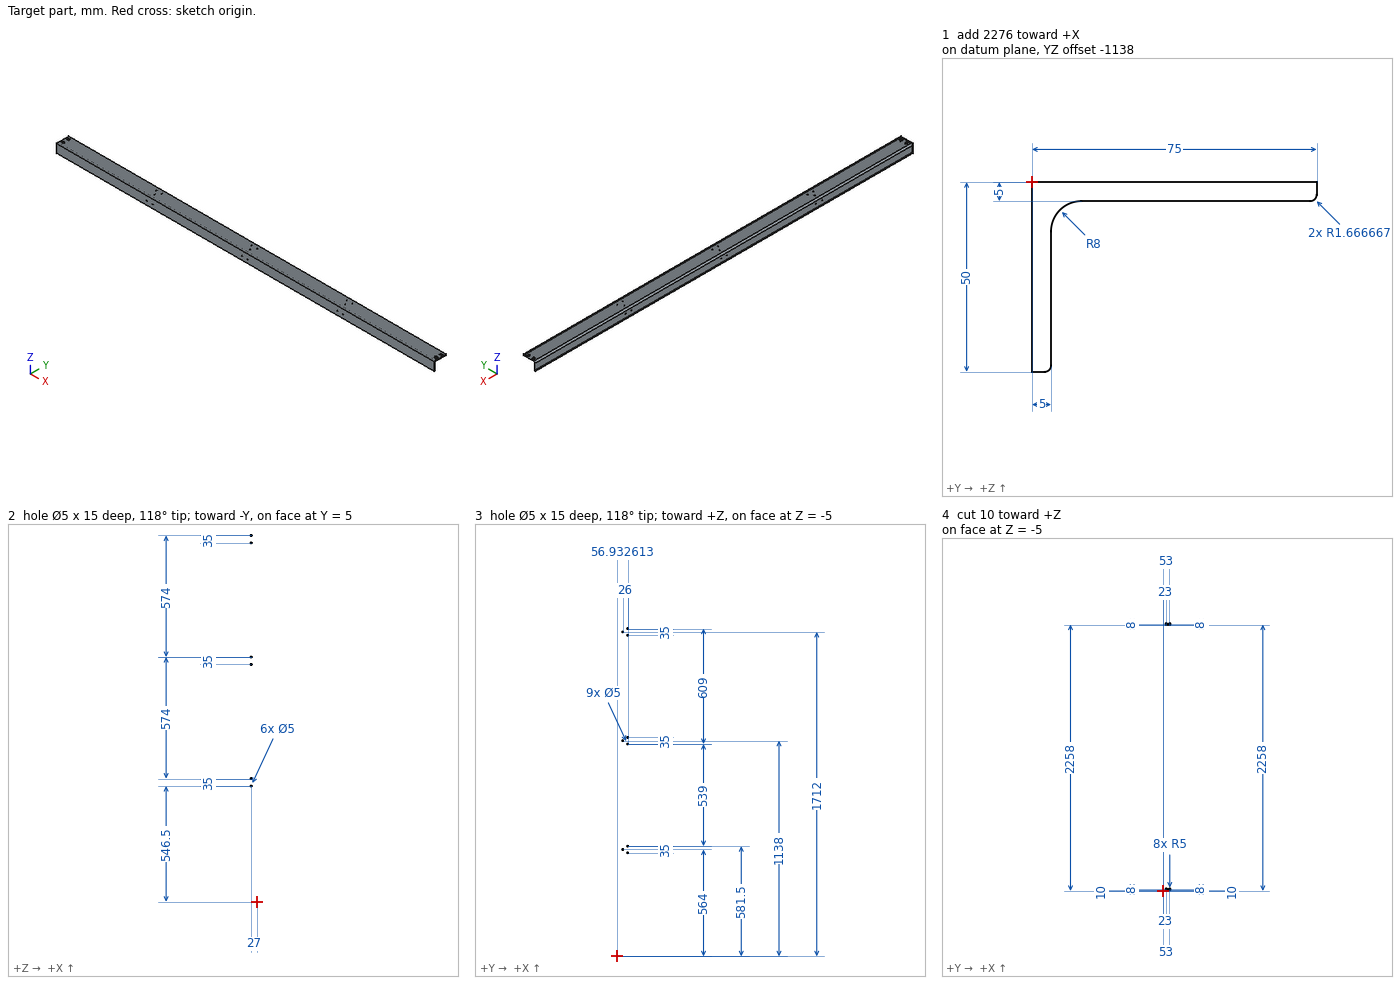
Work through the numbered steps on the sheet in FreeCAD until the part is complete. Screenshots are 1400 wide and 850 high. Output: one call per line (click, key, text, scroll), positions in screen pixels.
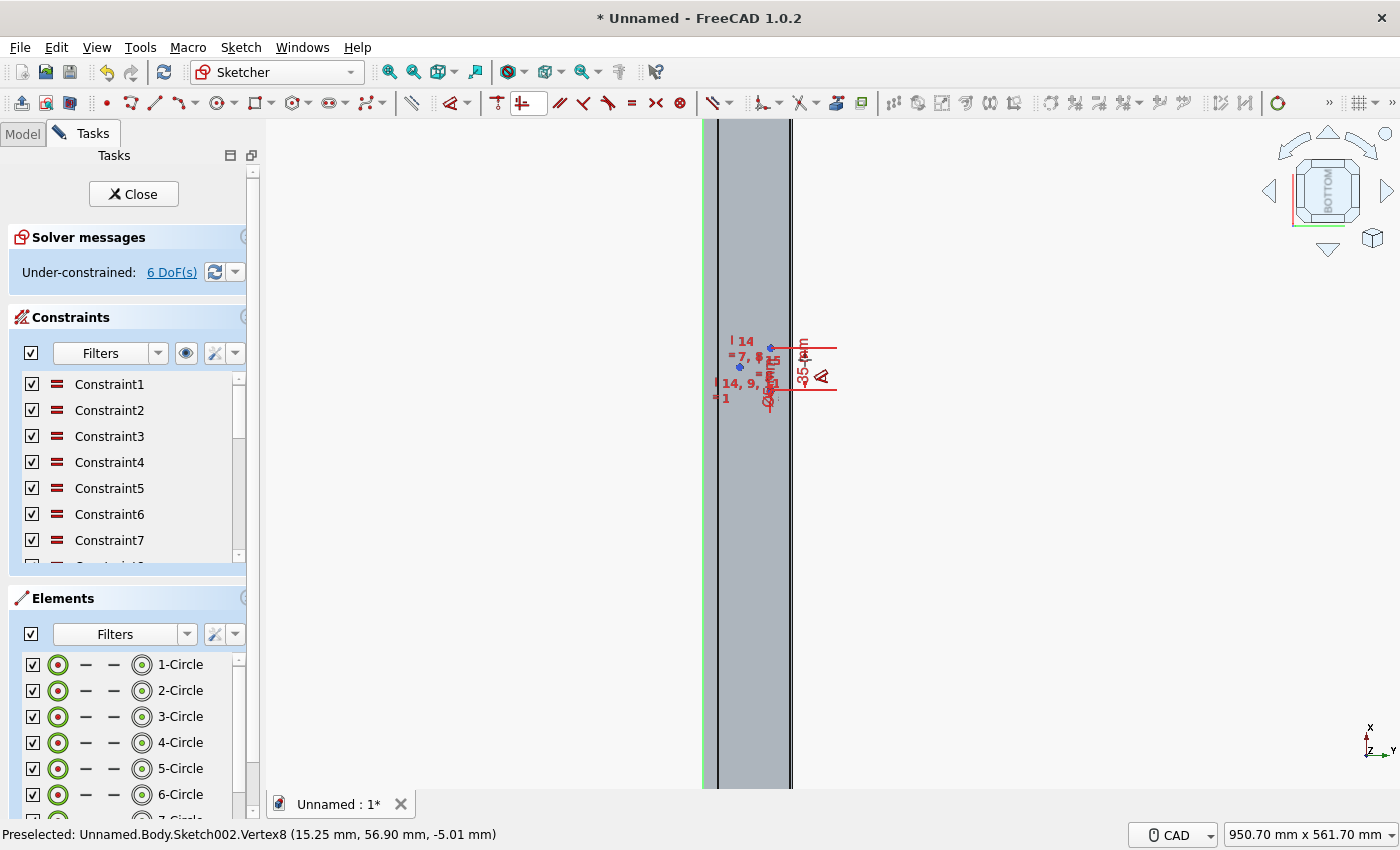
scroll(771, 394, down, 8)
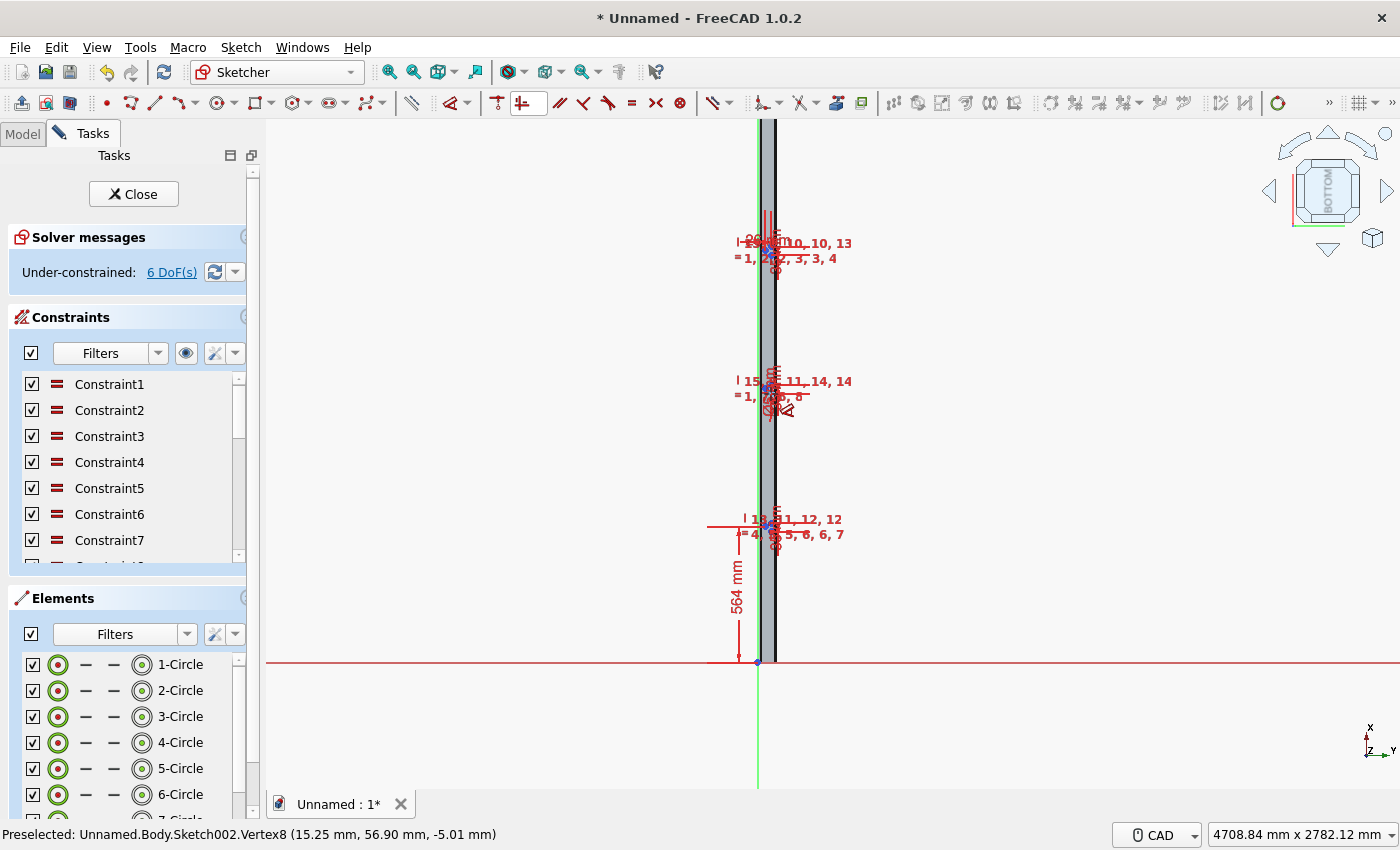
scroll(765, 251, up, 3)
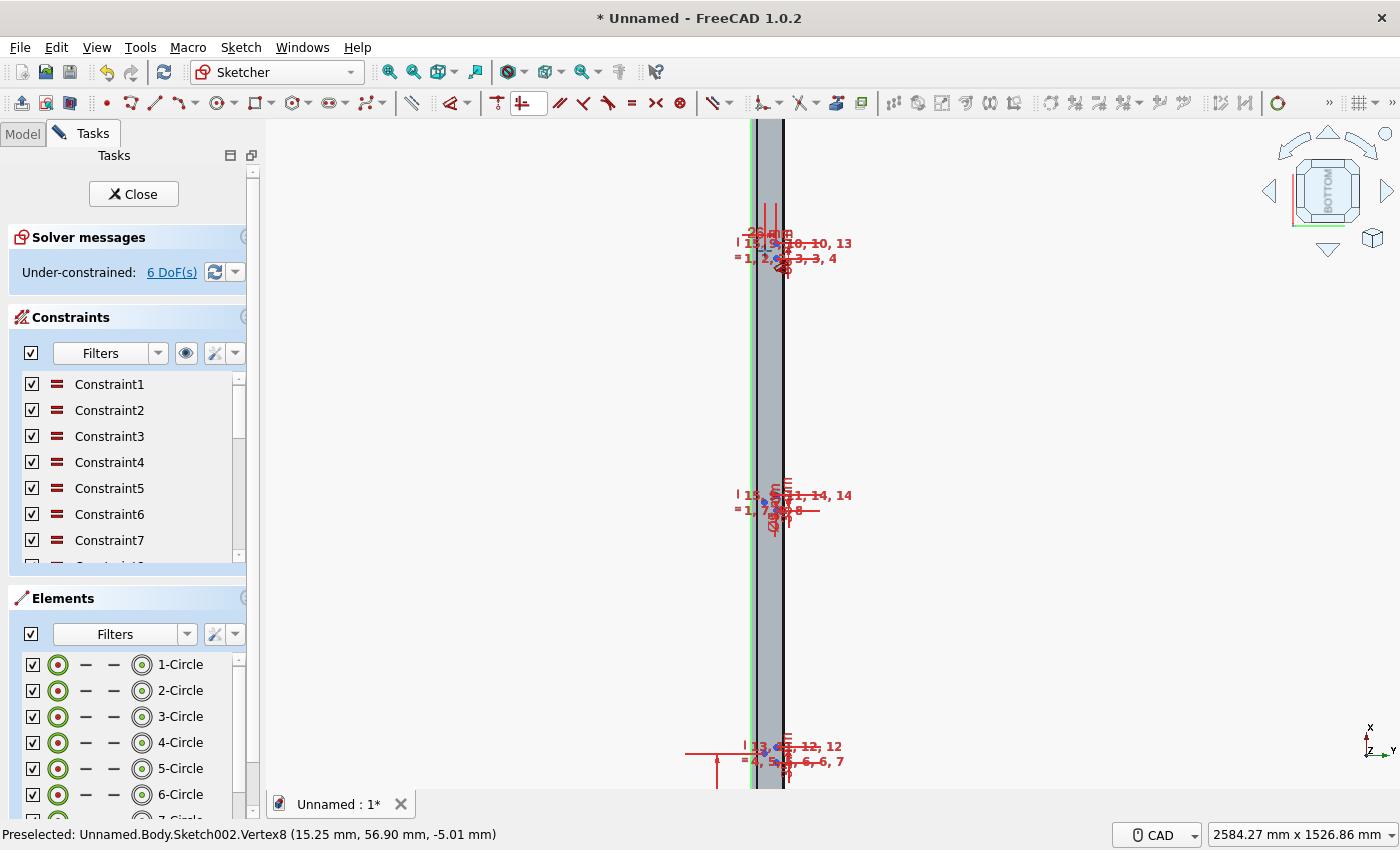
click(765, 250)
click(717, 388)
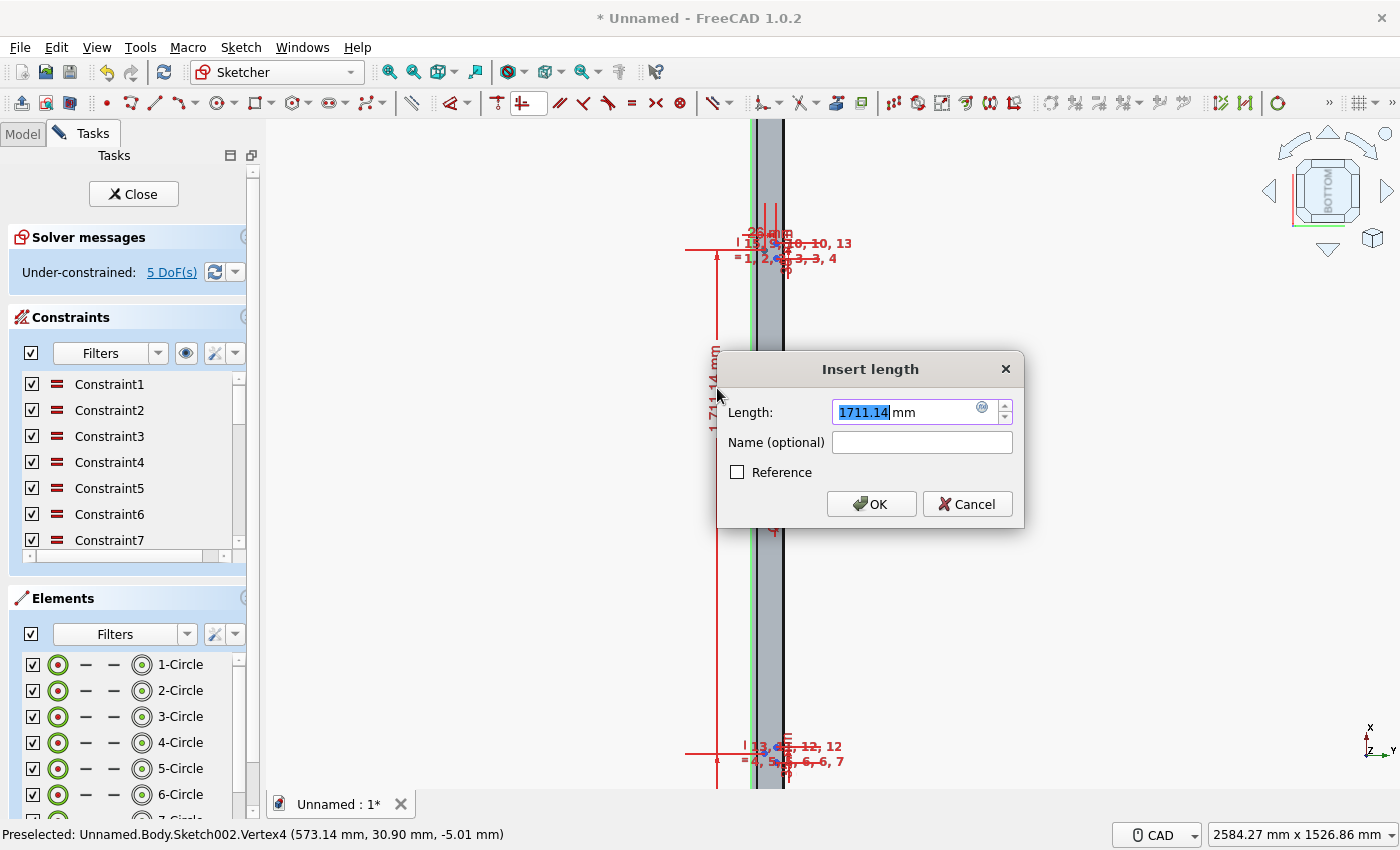
text(1712)
key(Return)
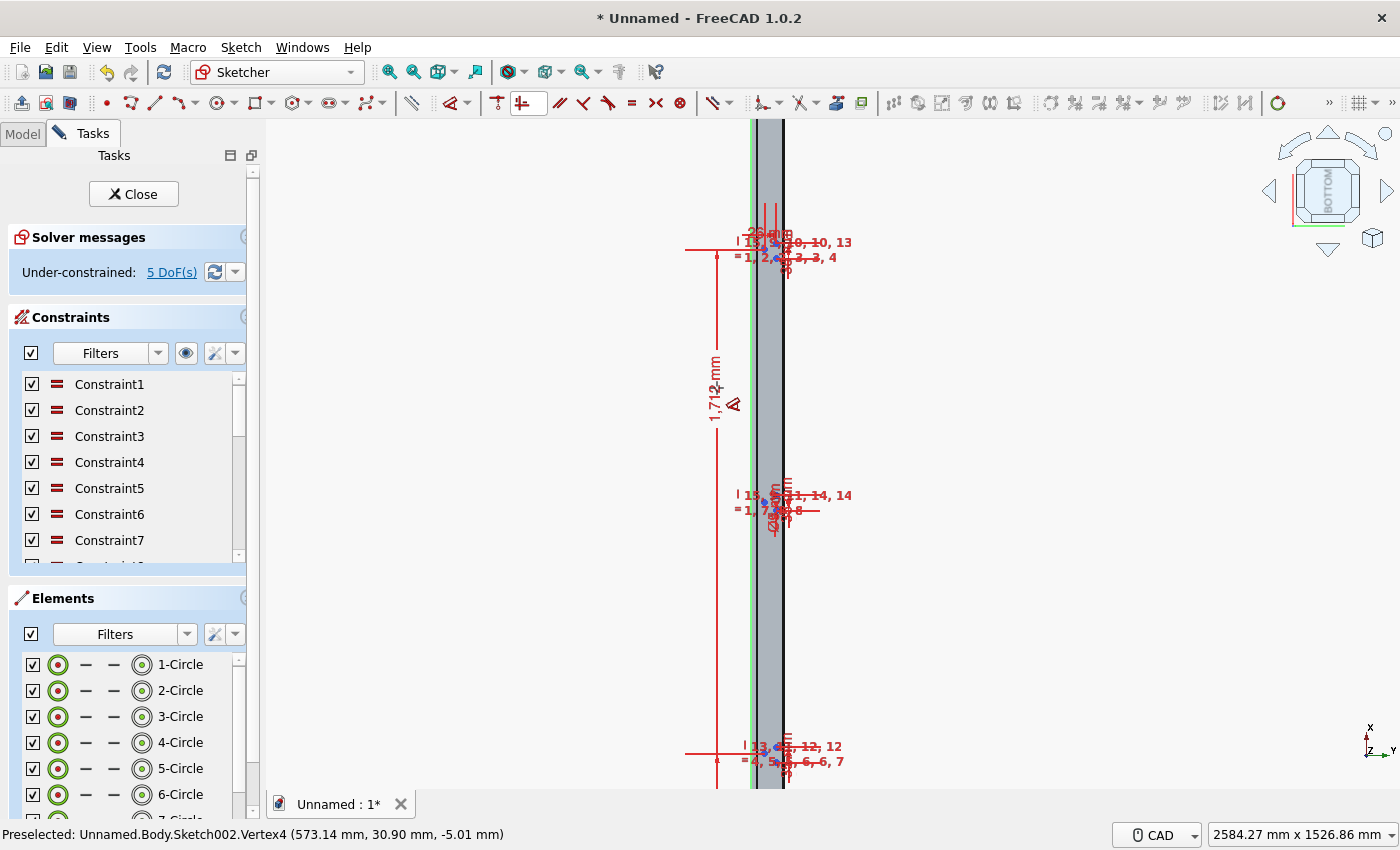
click(765, 502)
click(717, 632)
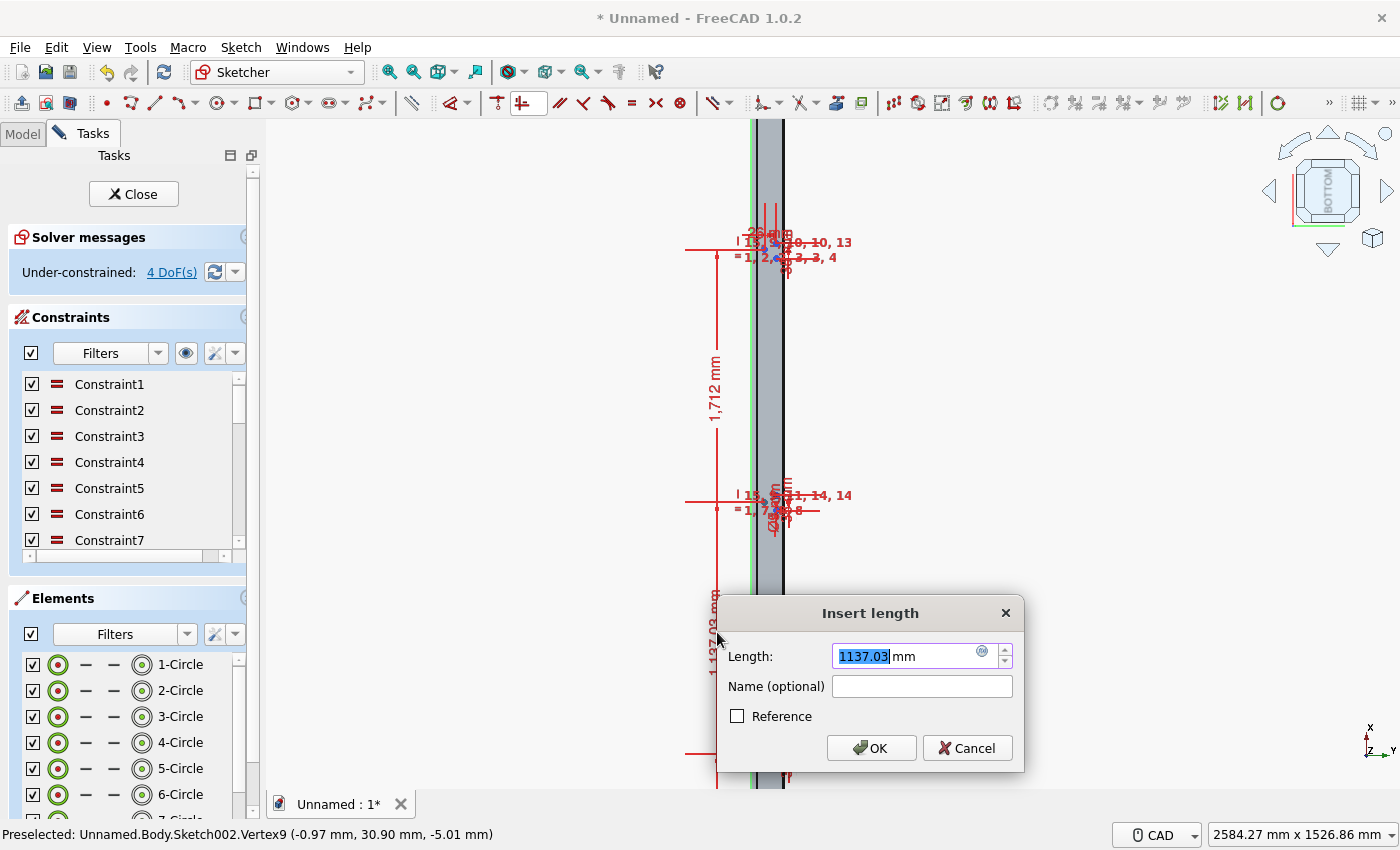
text(1138)
key(Return)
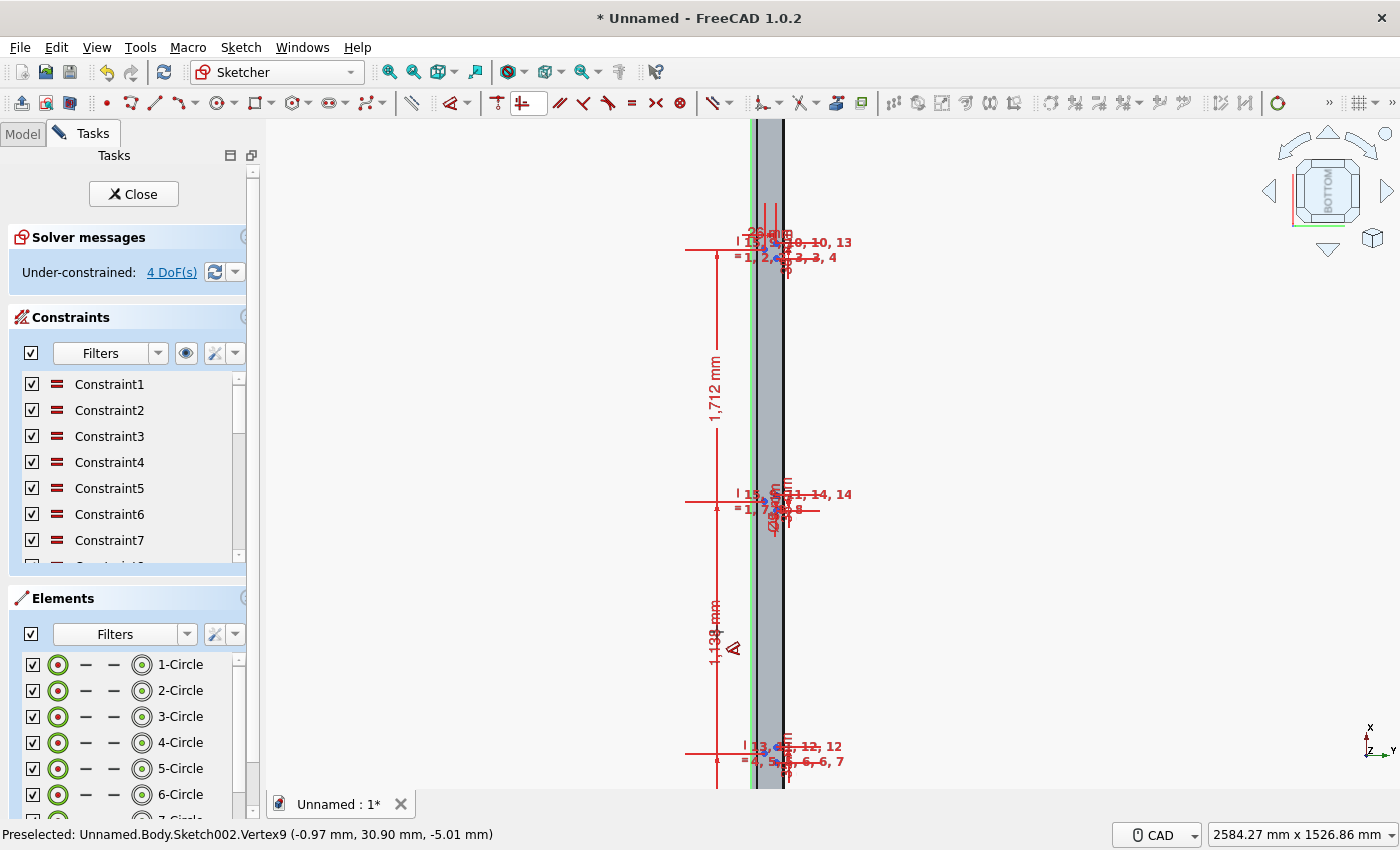
click(776, 511)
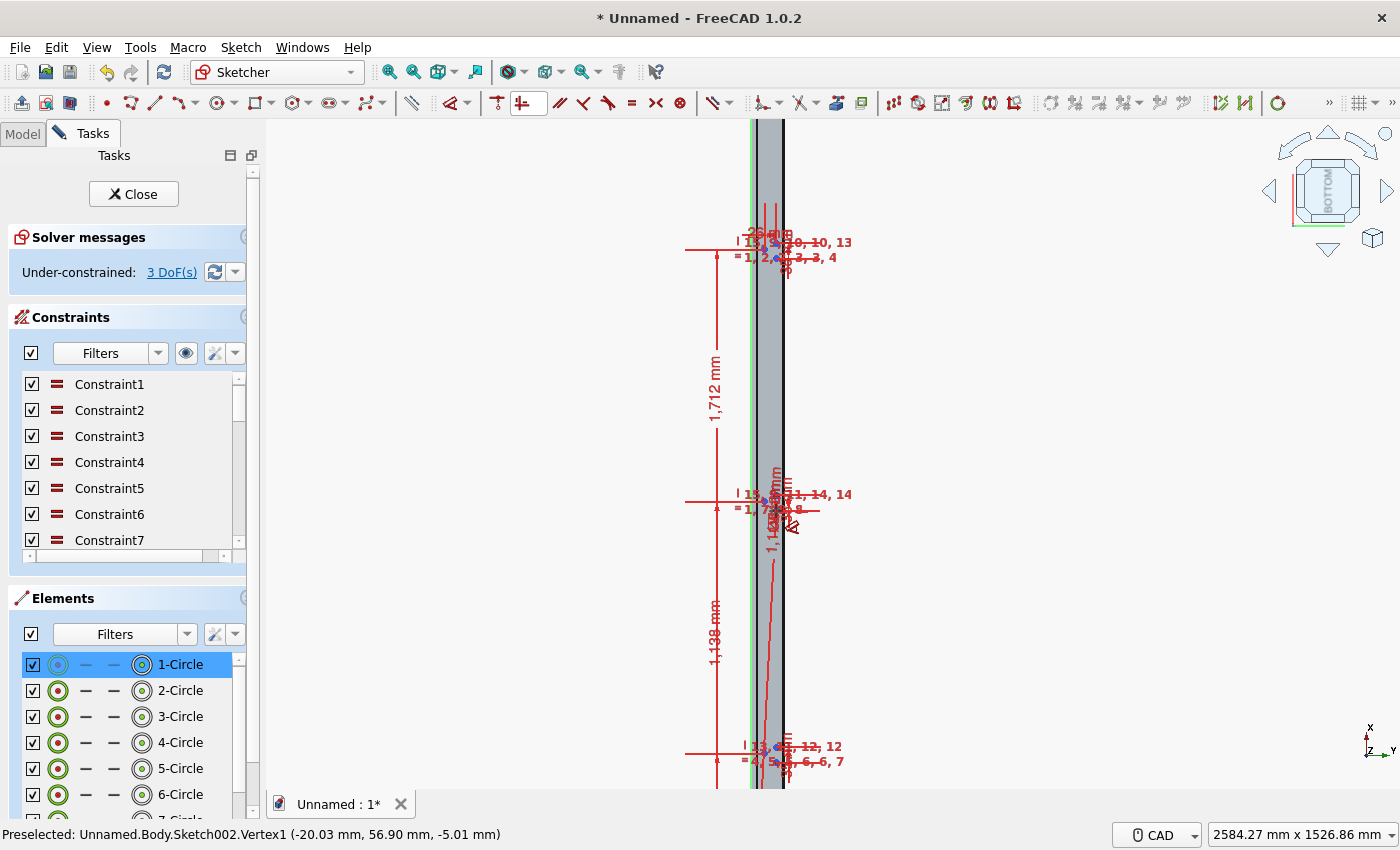
click(776, 243)
click(810, 377)